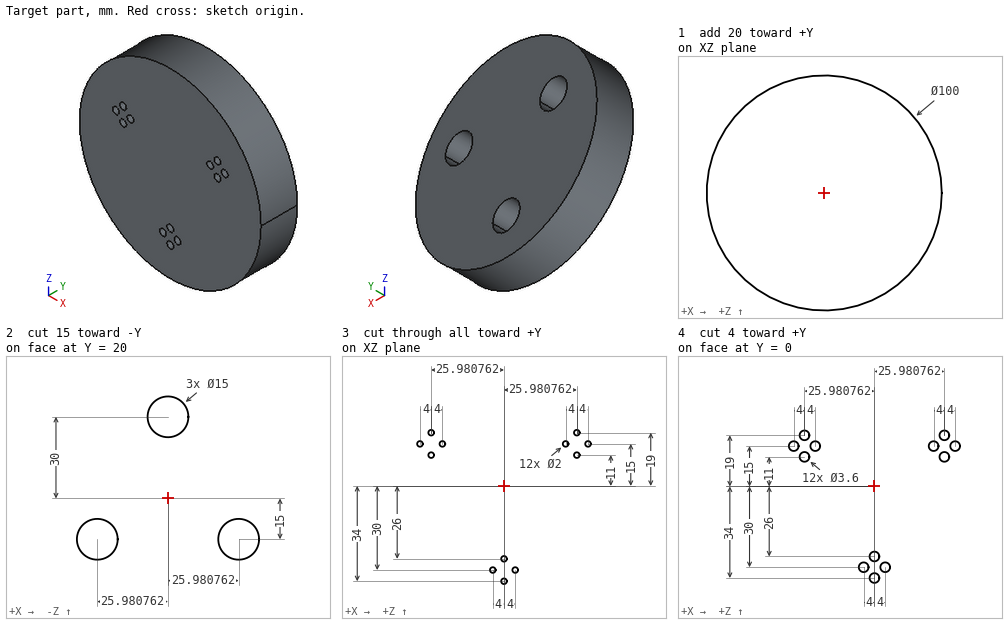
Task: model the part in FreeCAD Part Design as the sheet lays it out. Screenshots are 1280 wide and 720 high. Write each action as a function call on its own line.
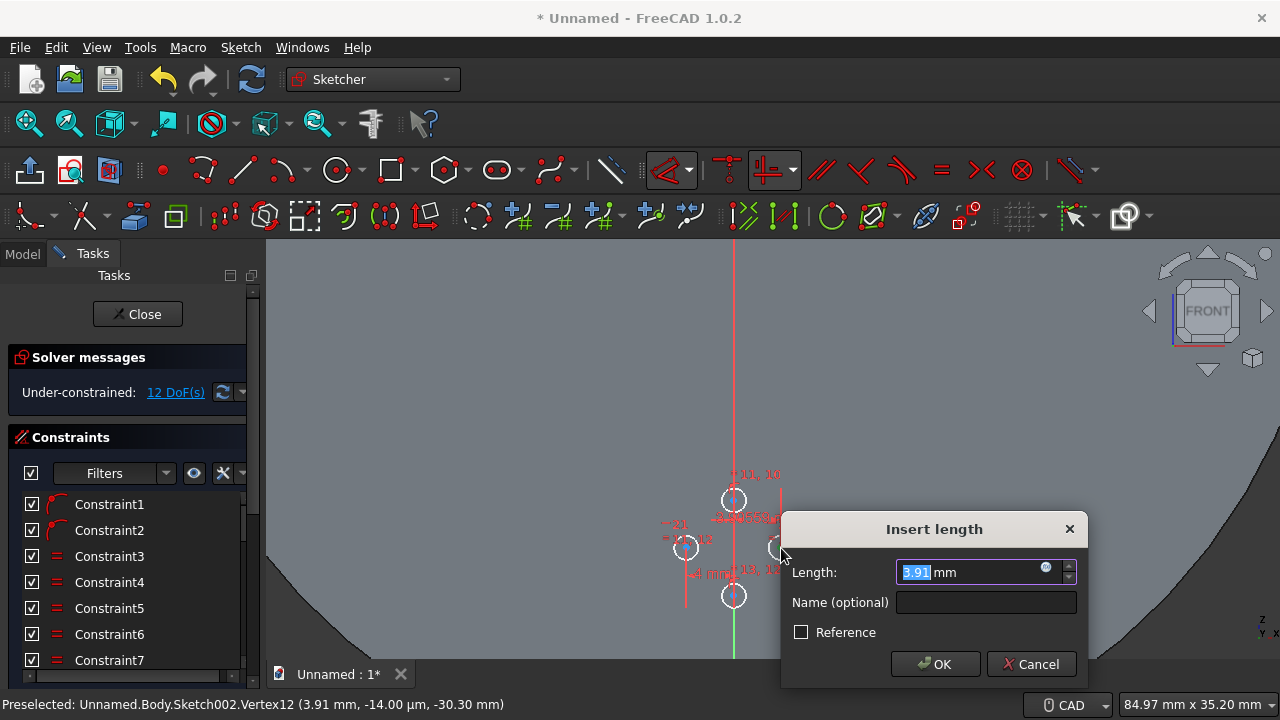
text(4)
key(Return)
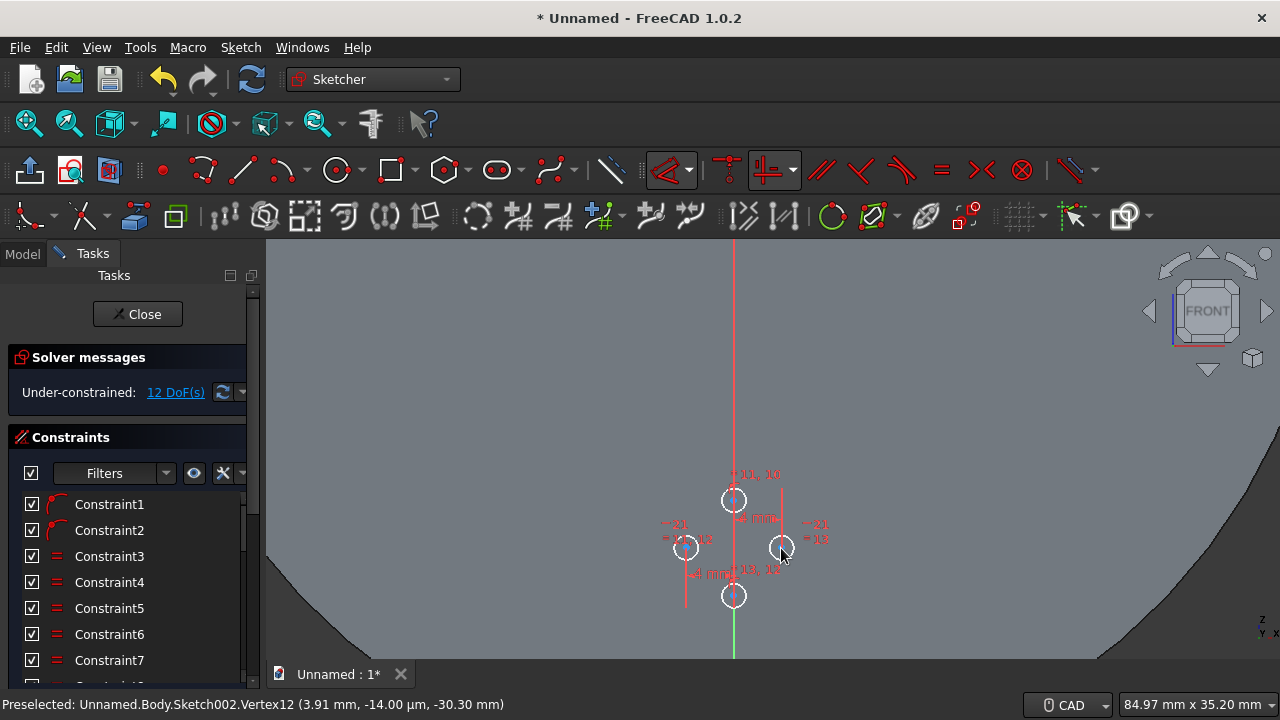
scroll(687, 550, down, 5)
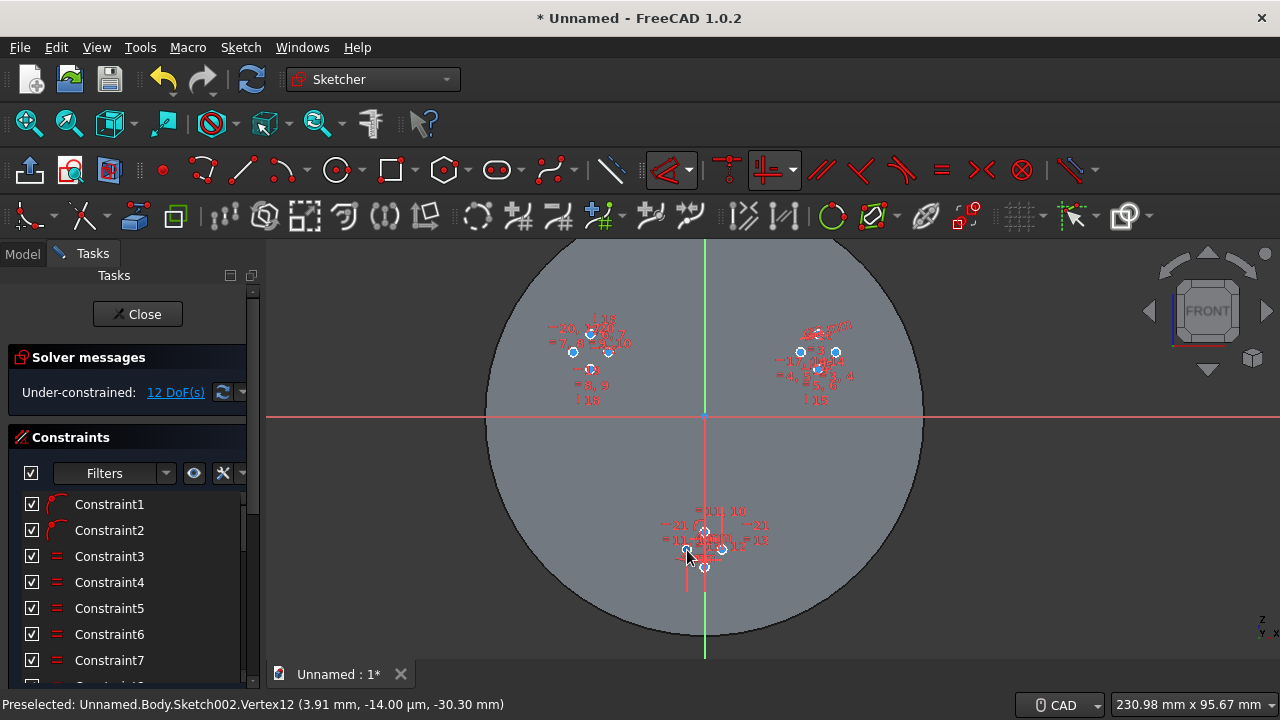
click(818, 334)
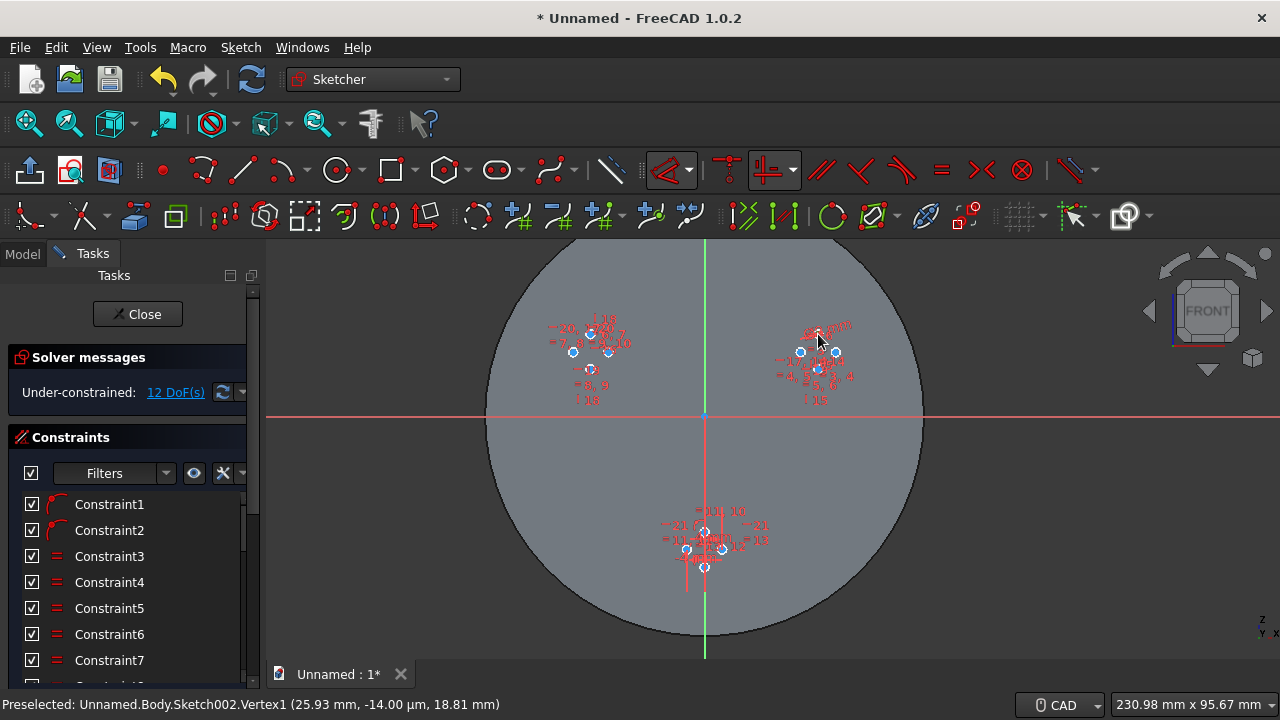
click(692, 170)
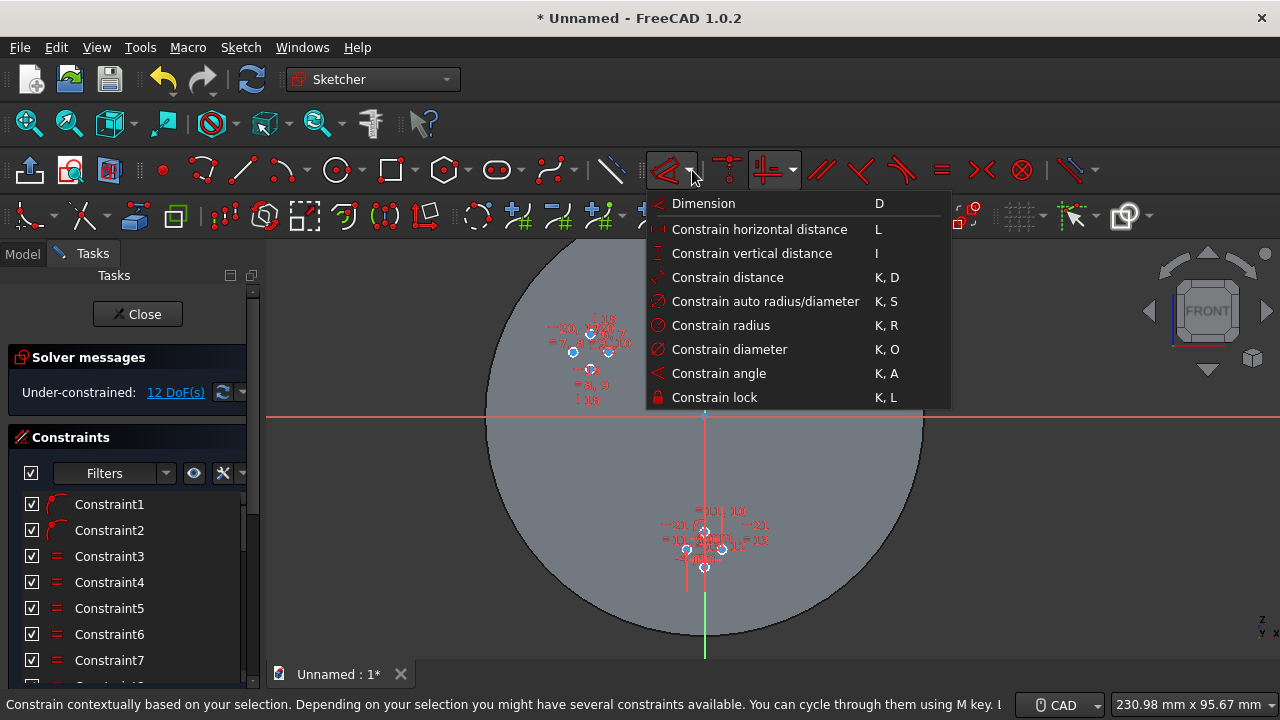
click(799, 253)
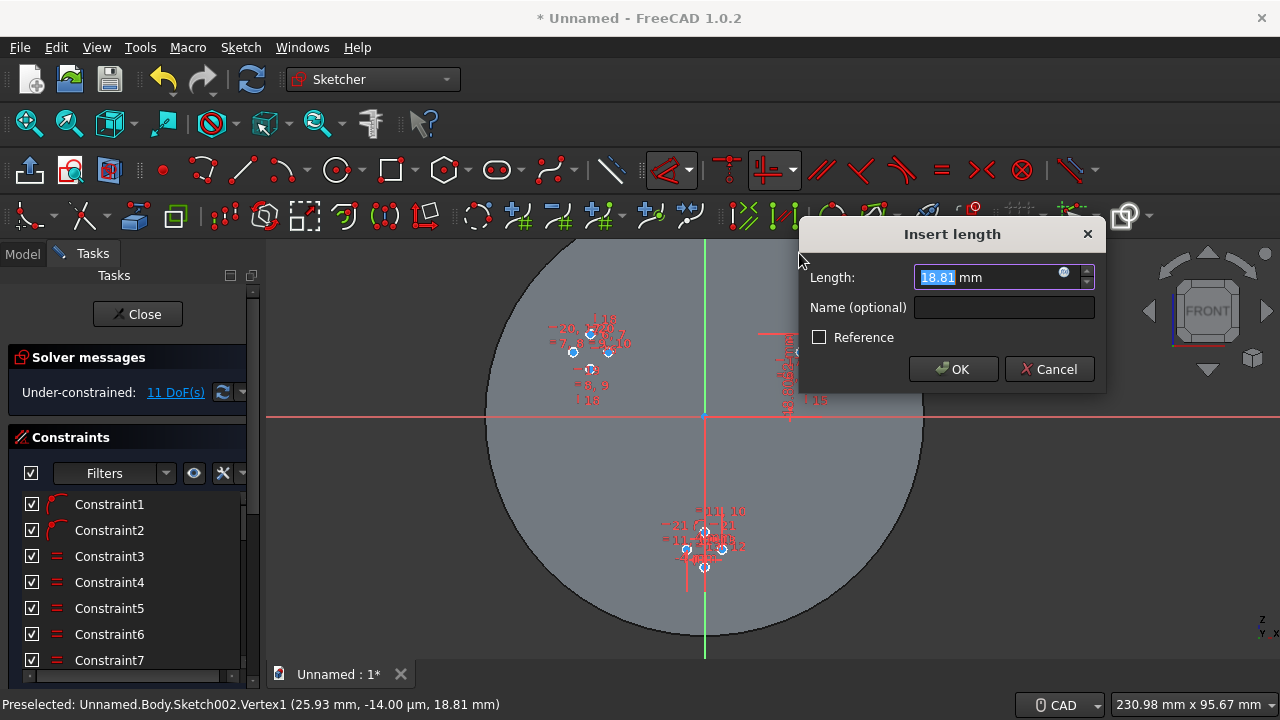
text(19)
key(Return)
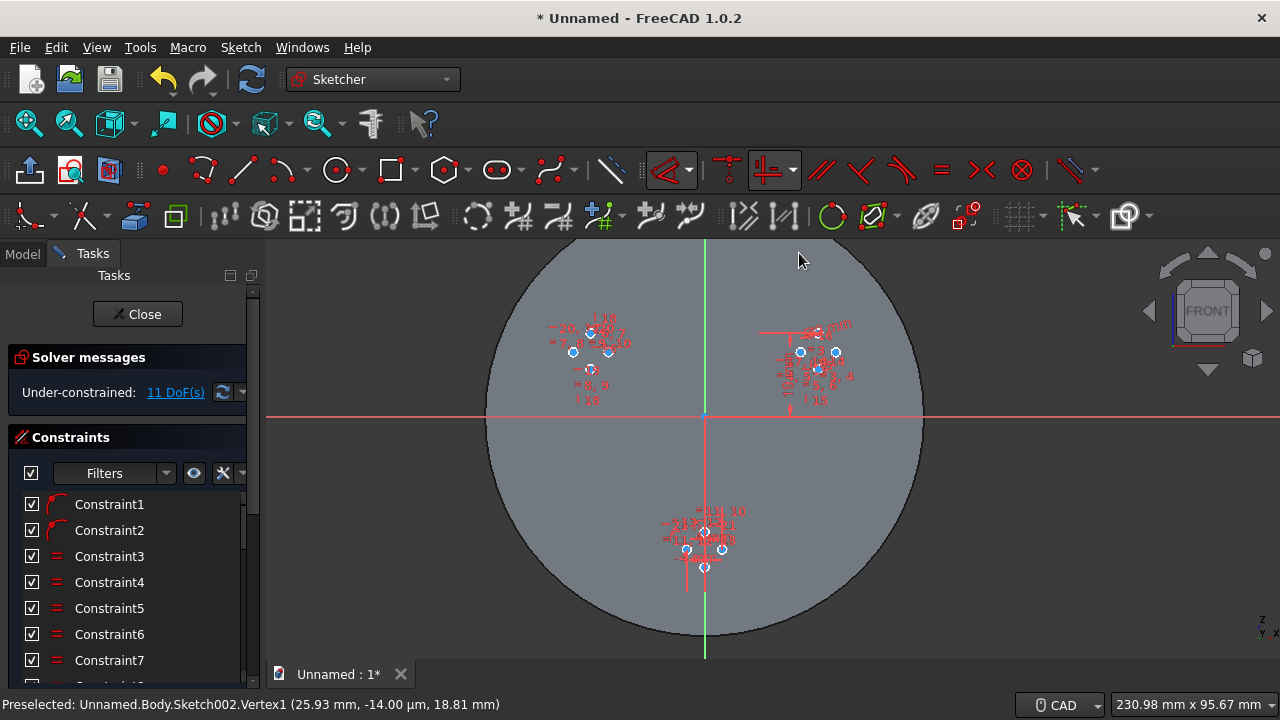
click(836, 352)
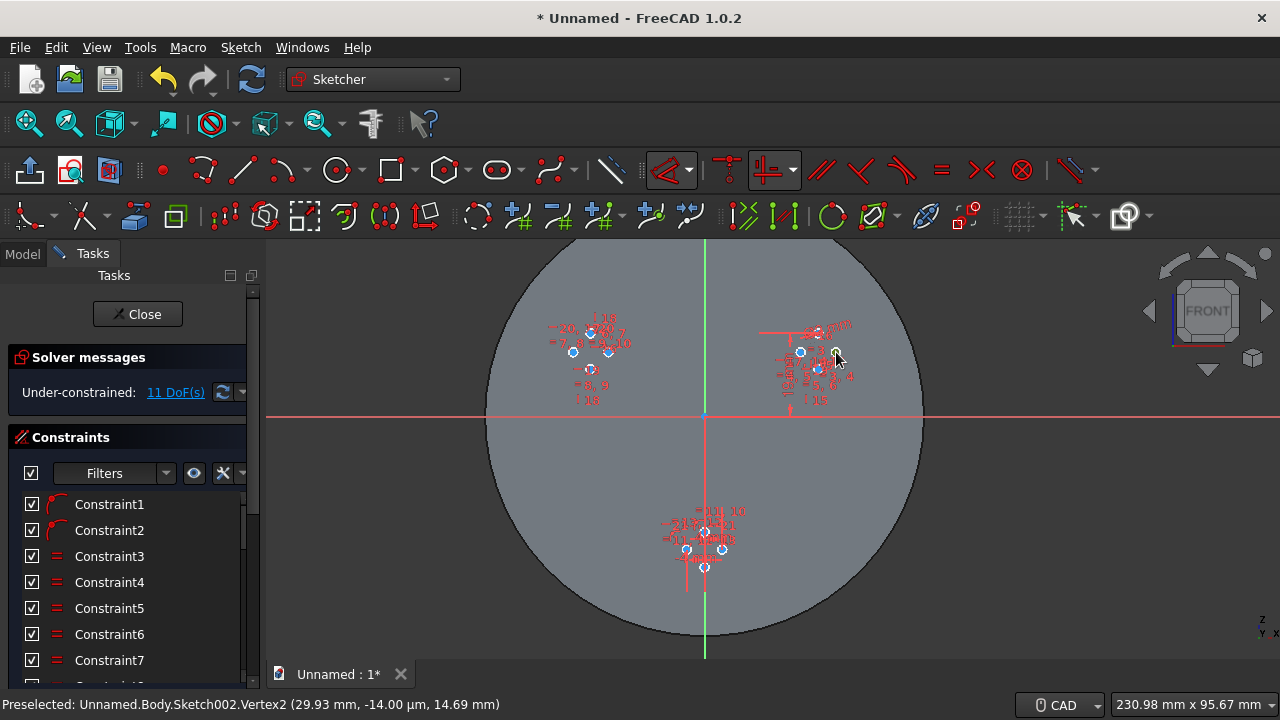
click(692, 170)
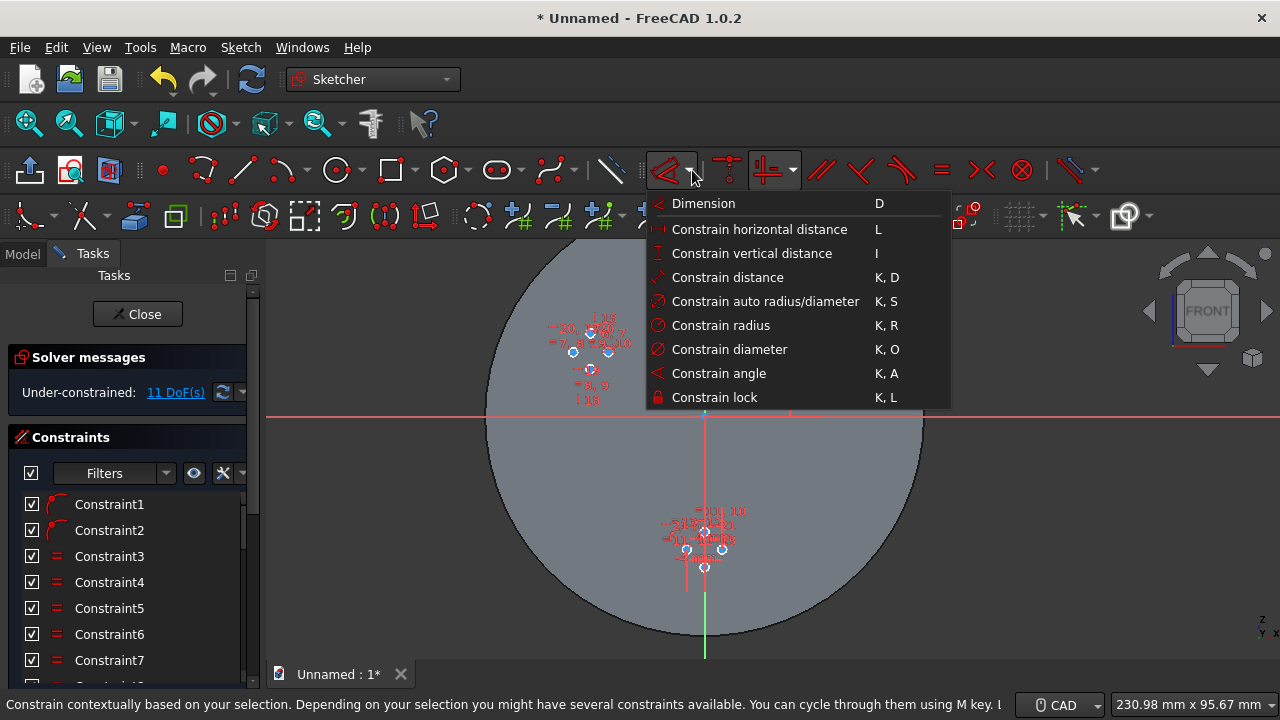
click(799, 253)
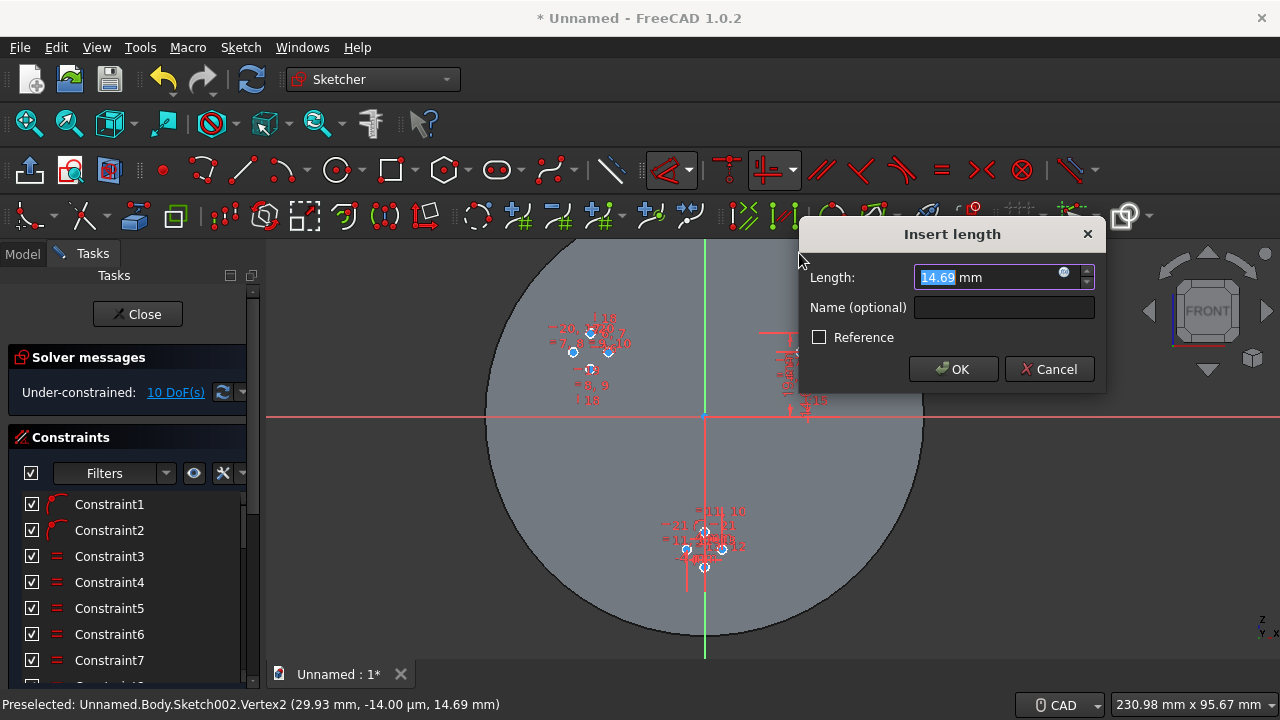
text(15)
key(Return)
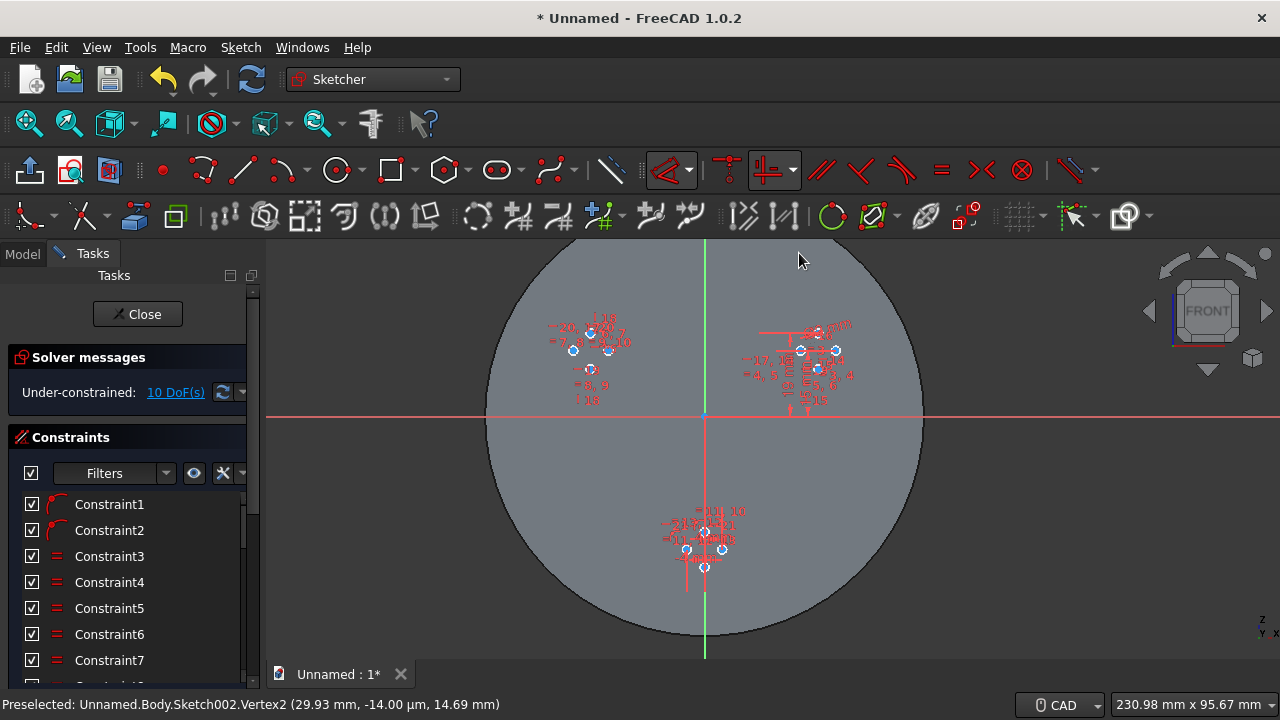
click(818, 369)